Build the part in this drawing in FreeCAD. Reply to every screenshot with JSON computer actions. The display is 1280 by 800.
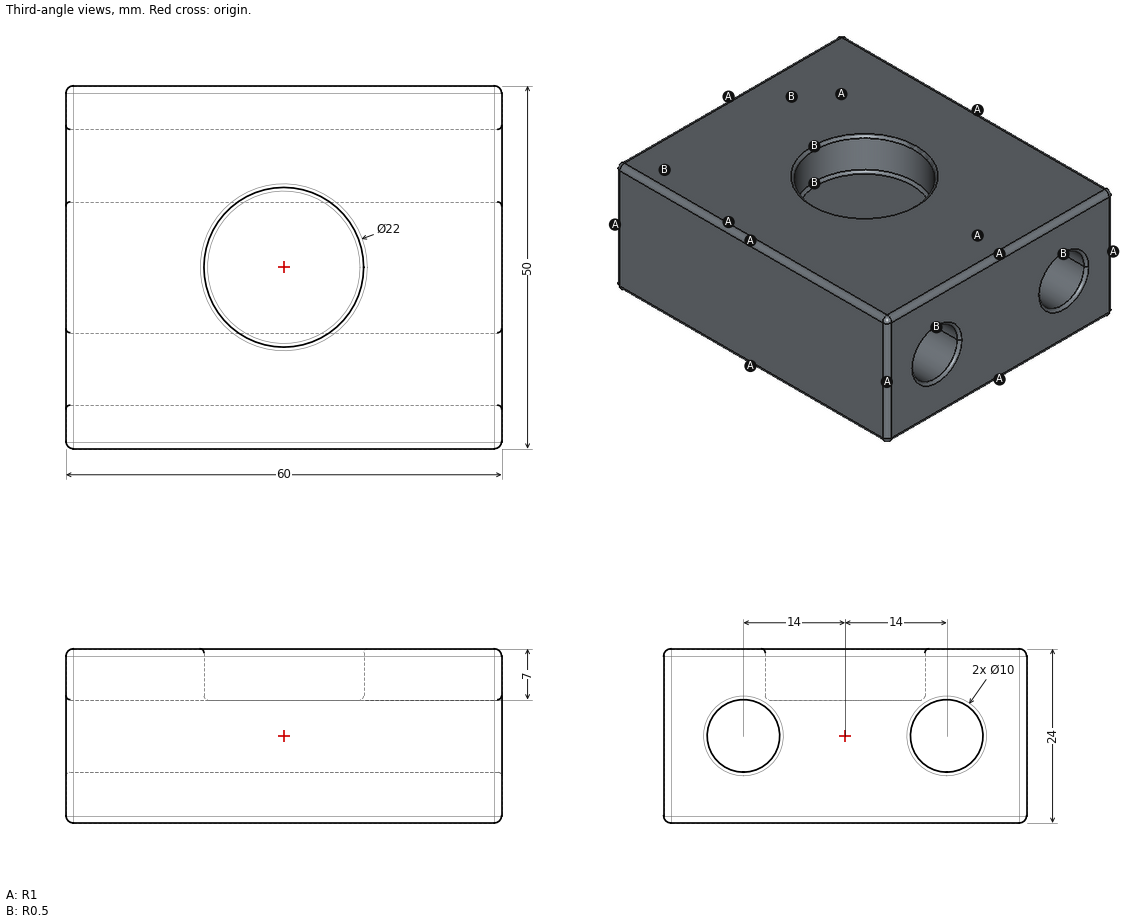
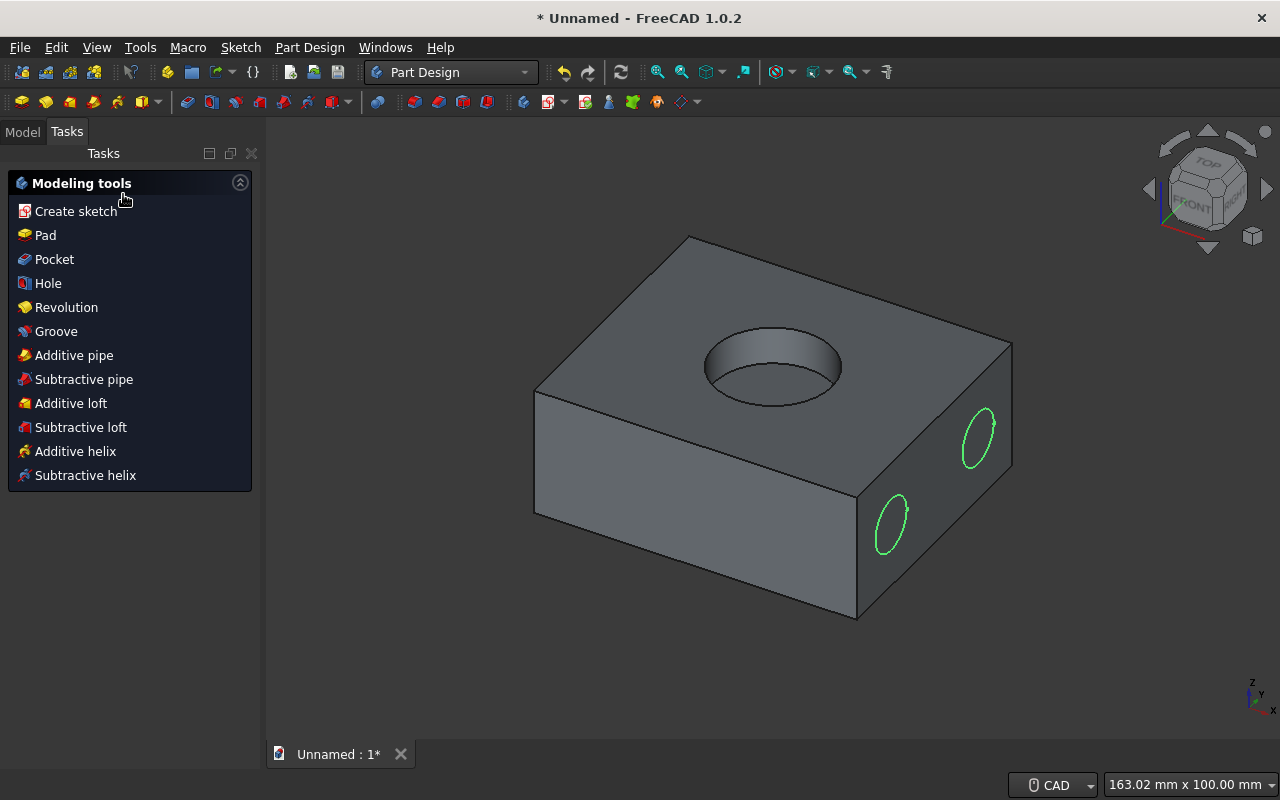
{"action": "left_click", "coordinate": [188, 102]}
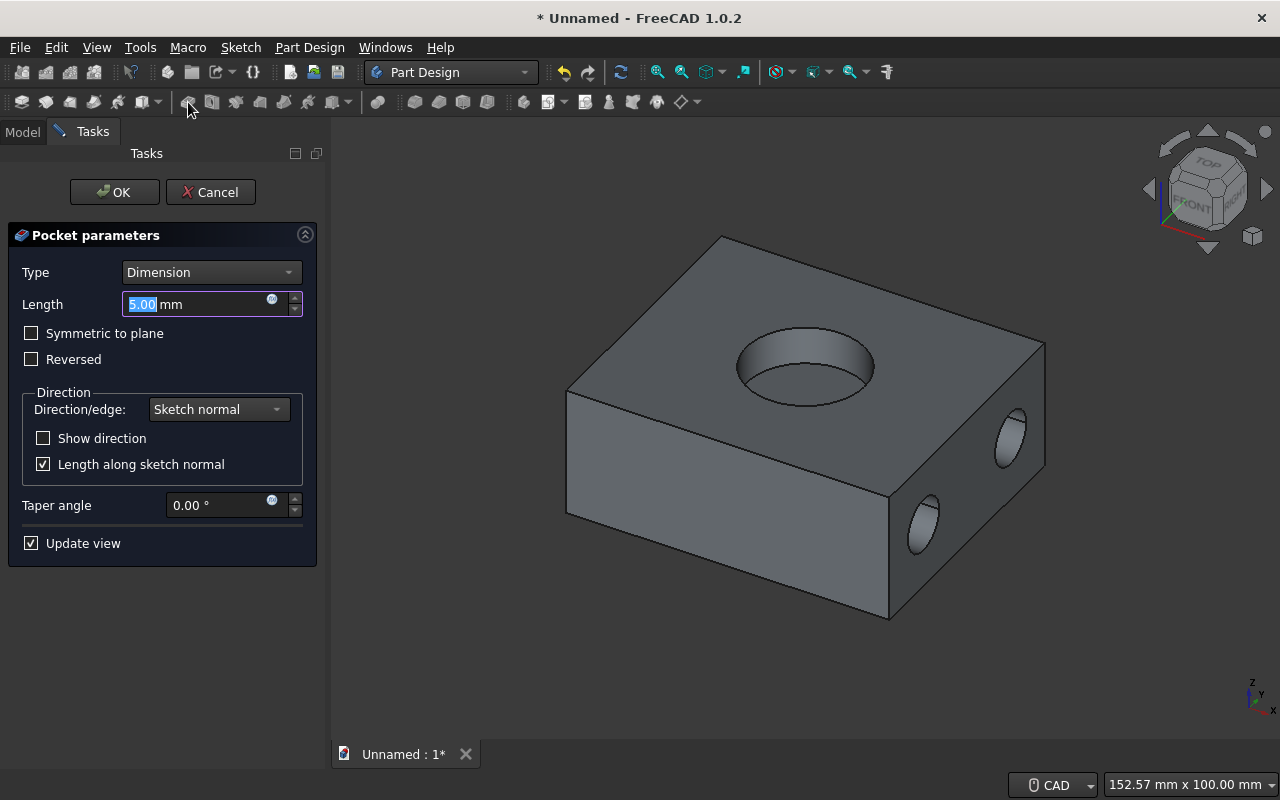
{"action": "left_click", "coordinate": [212, 272]}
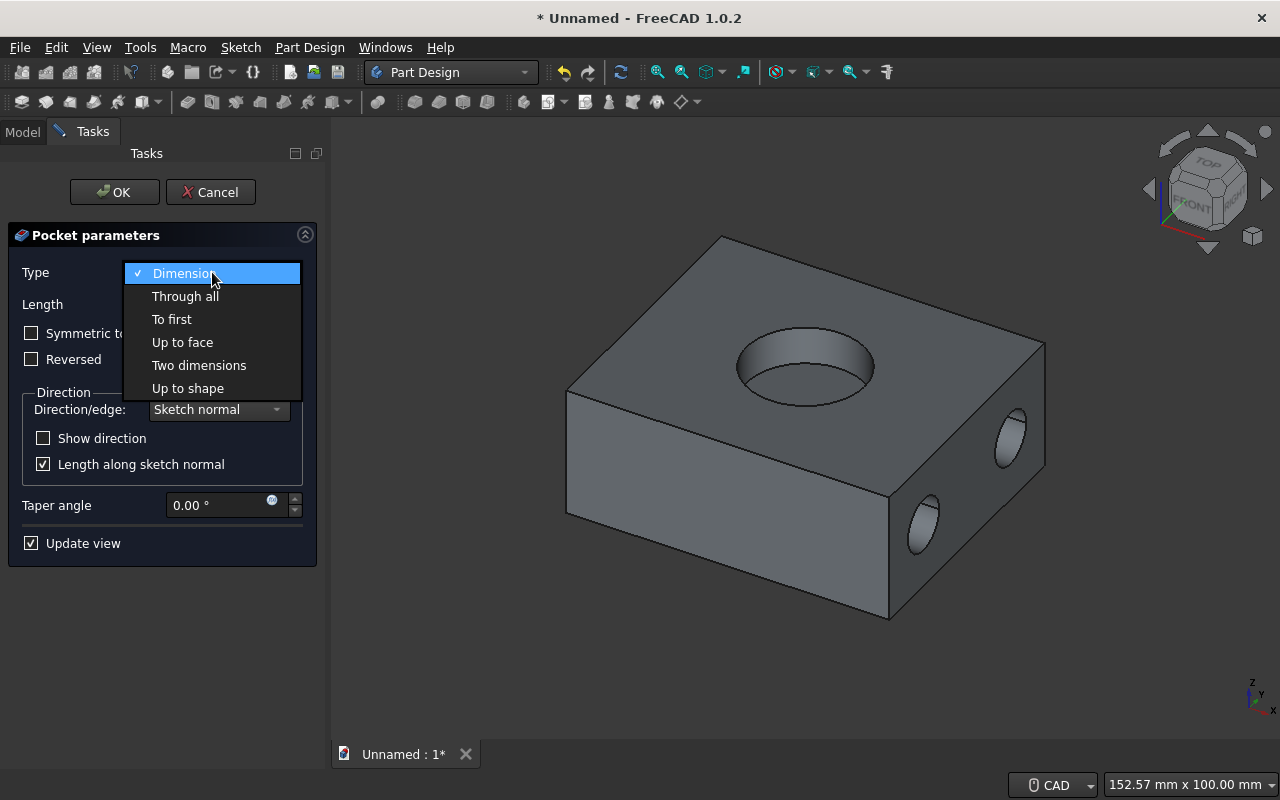
{"action": "left_click", "coordinate": [212, 296]}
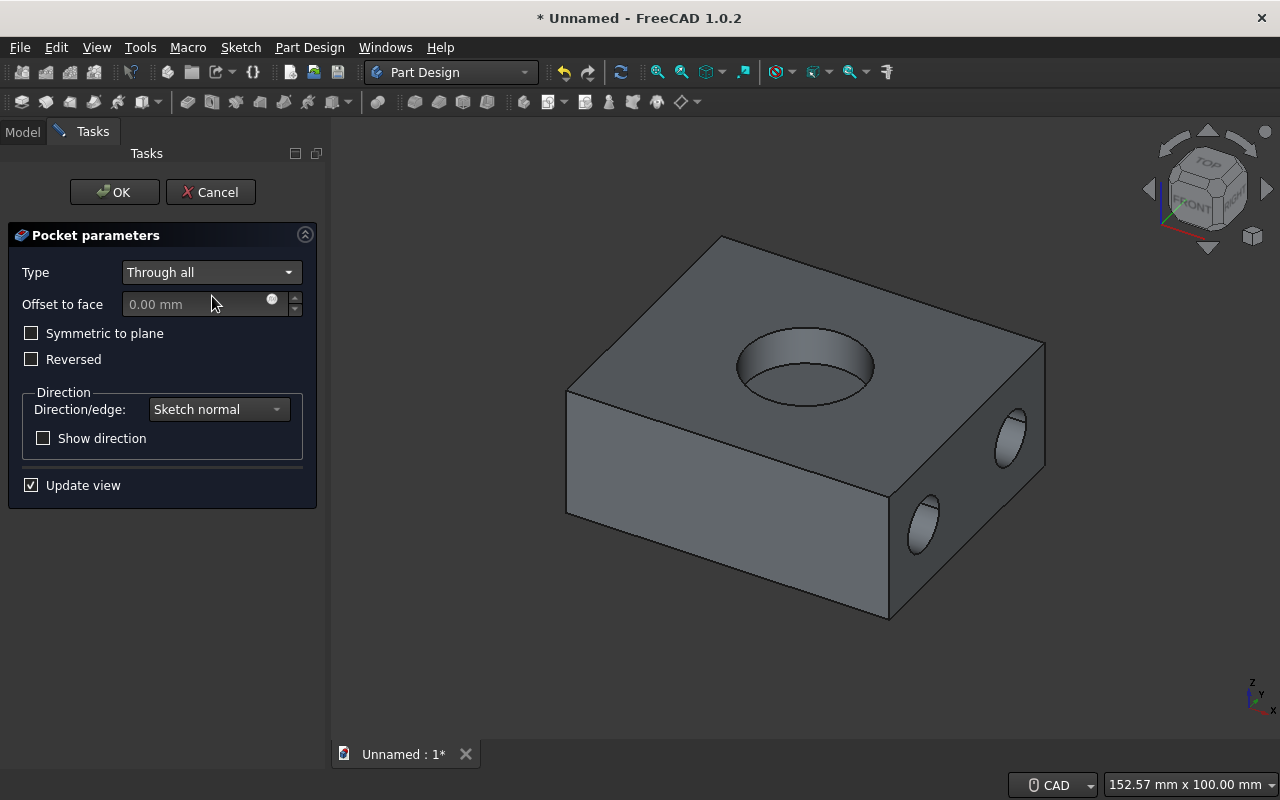
{"action": "left_click", "coordinate": [115, 192]}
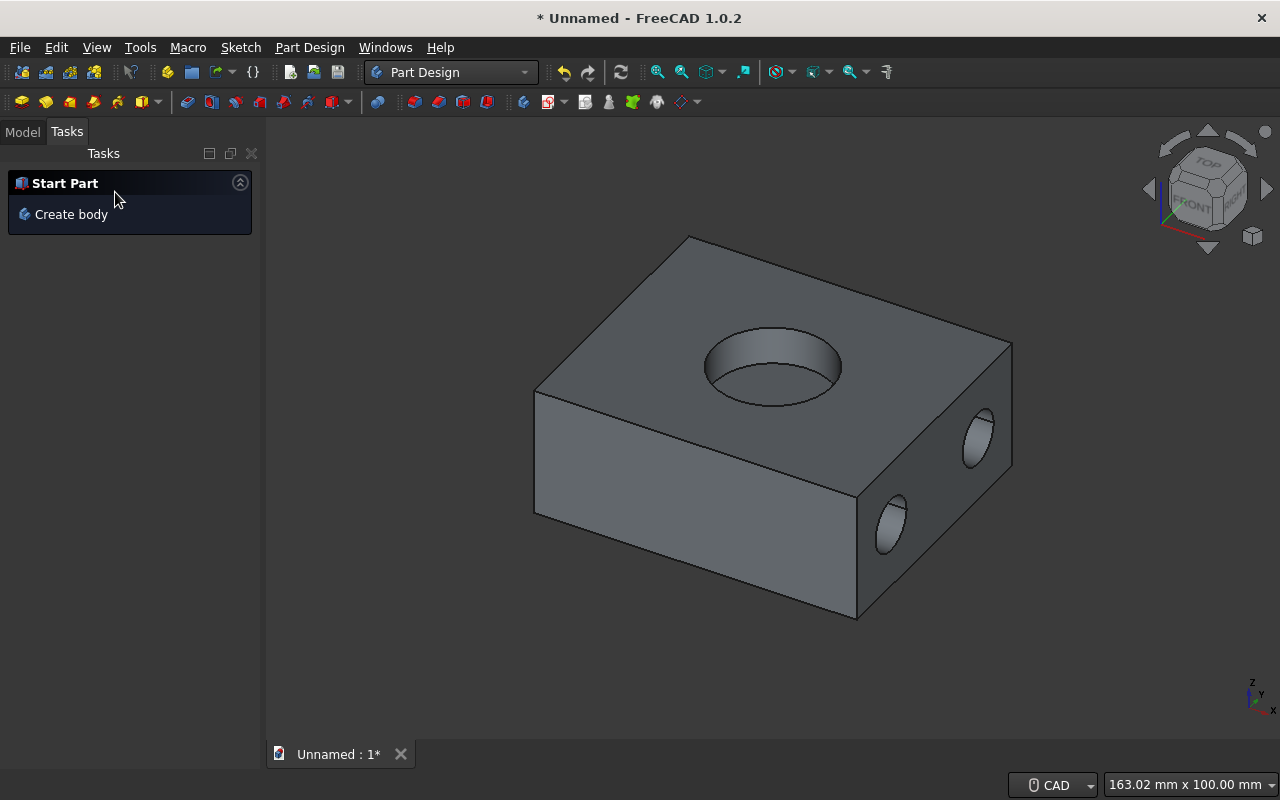
{"action": "left_click", "coordinate": [788, 535]}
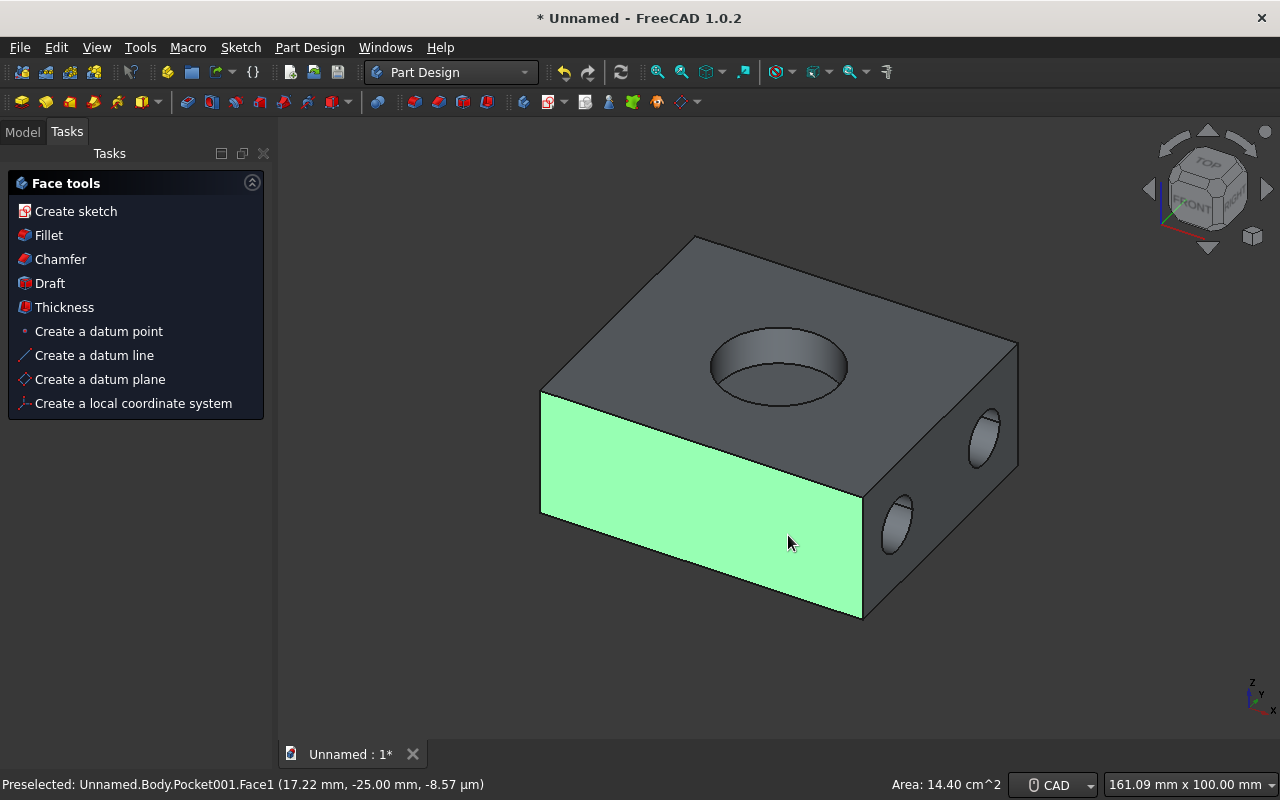
{"action": "left_click", "coordinate": [941, 419], "text": "ctrl"}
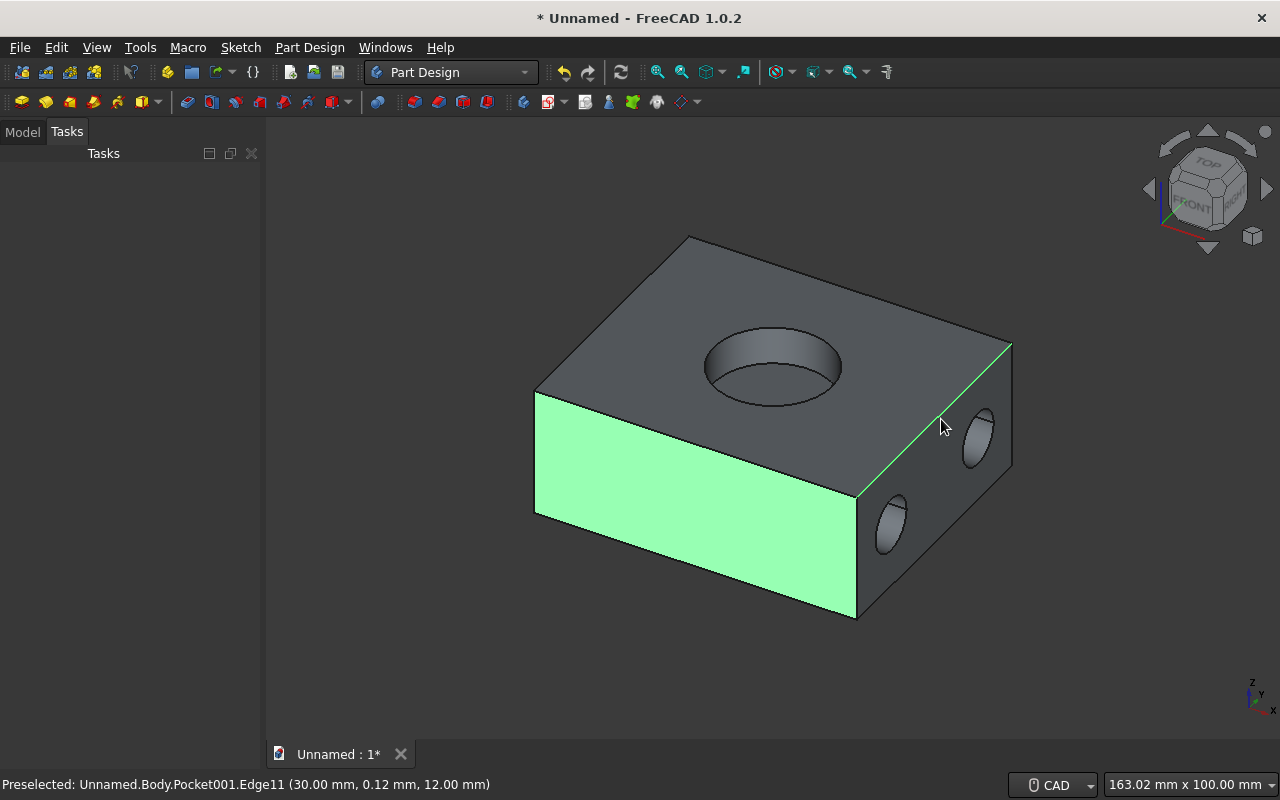
{"action": "key", "text": "0"}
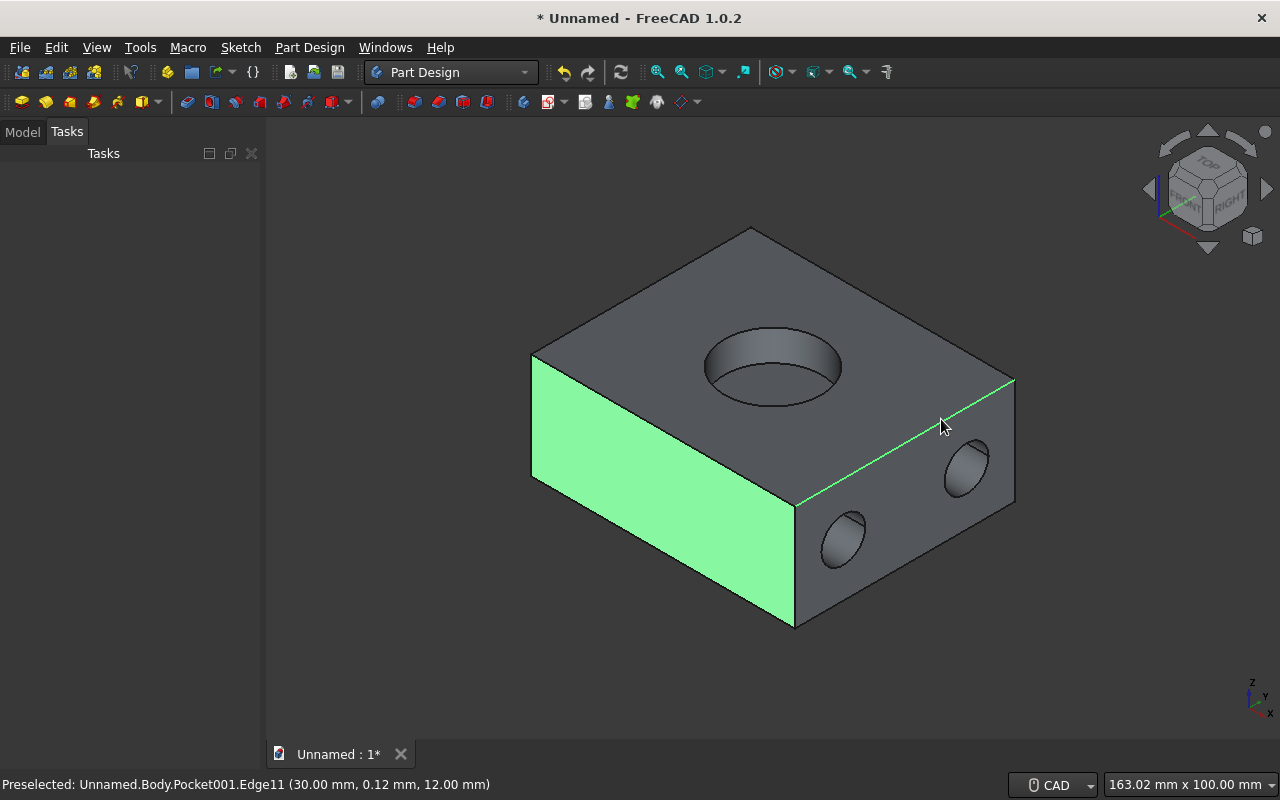
{"action": "key", "text": "2"}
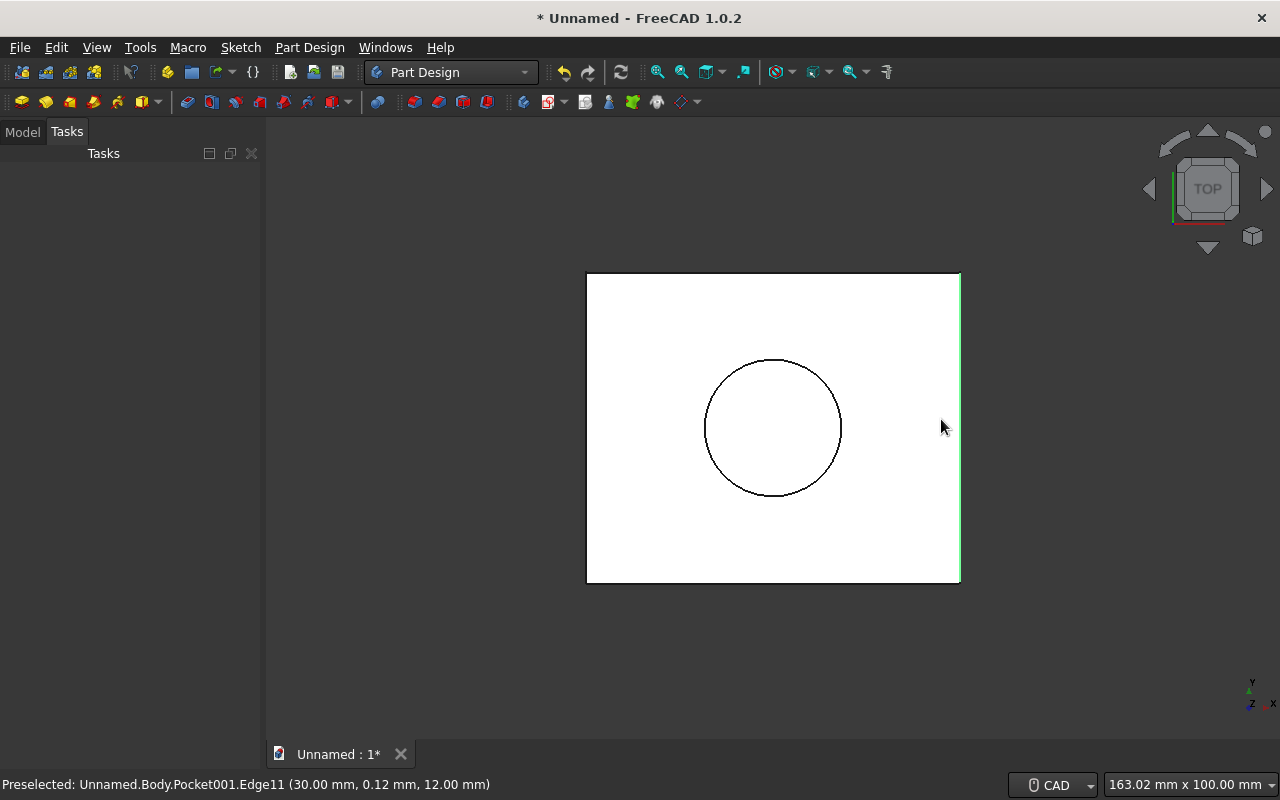
{"action": "left_click", "coordinate": [586, 427], "text": "ctrl"}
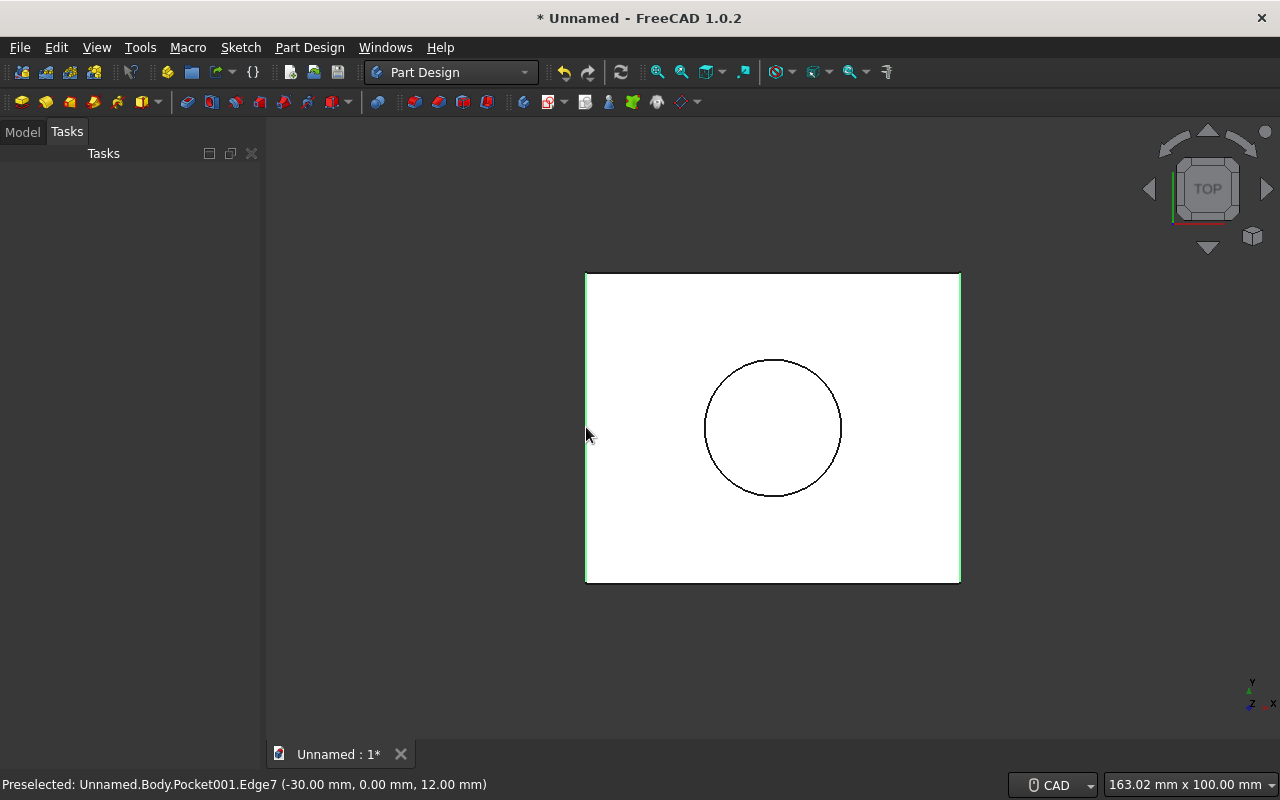
{"action": "key", "text": "1"}